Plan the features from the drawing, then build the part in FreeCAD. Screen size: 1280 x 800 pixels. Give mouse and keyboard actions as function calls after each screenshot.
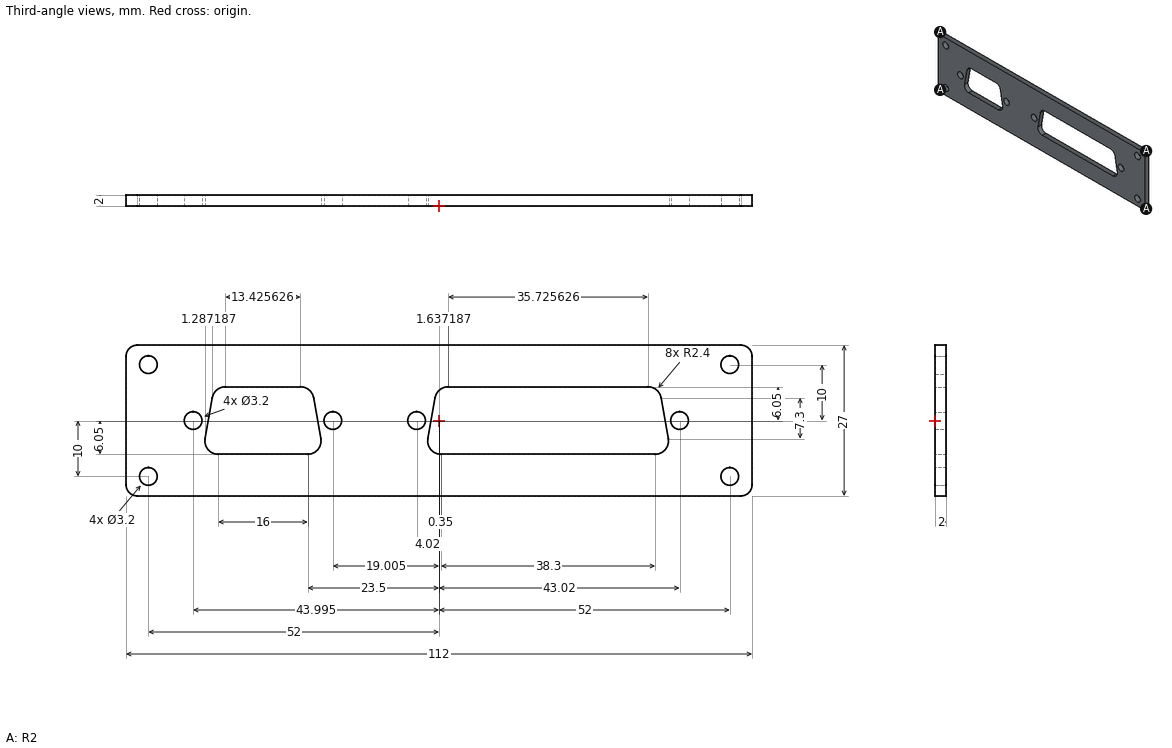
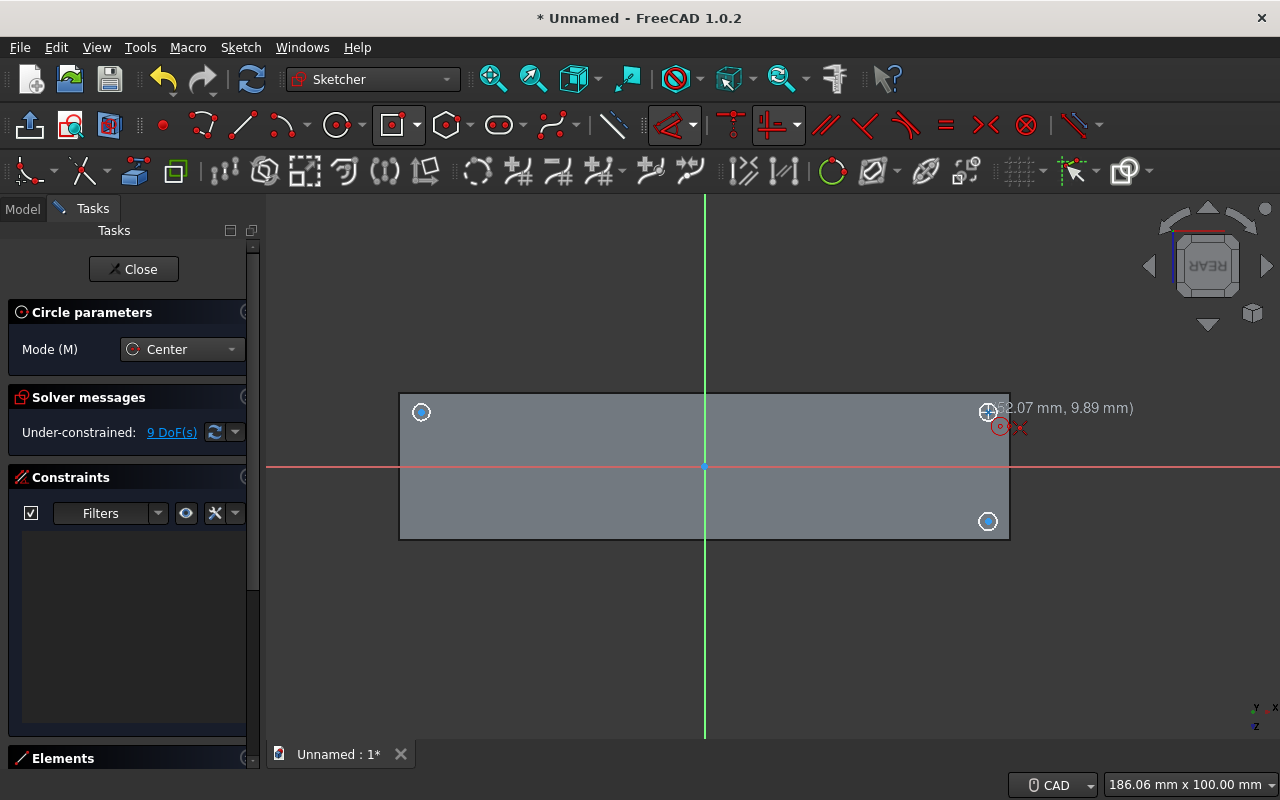
scroll(421, 521, up, 5)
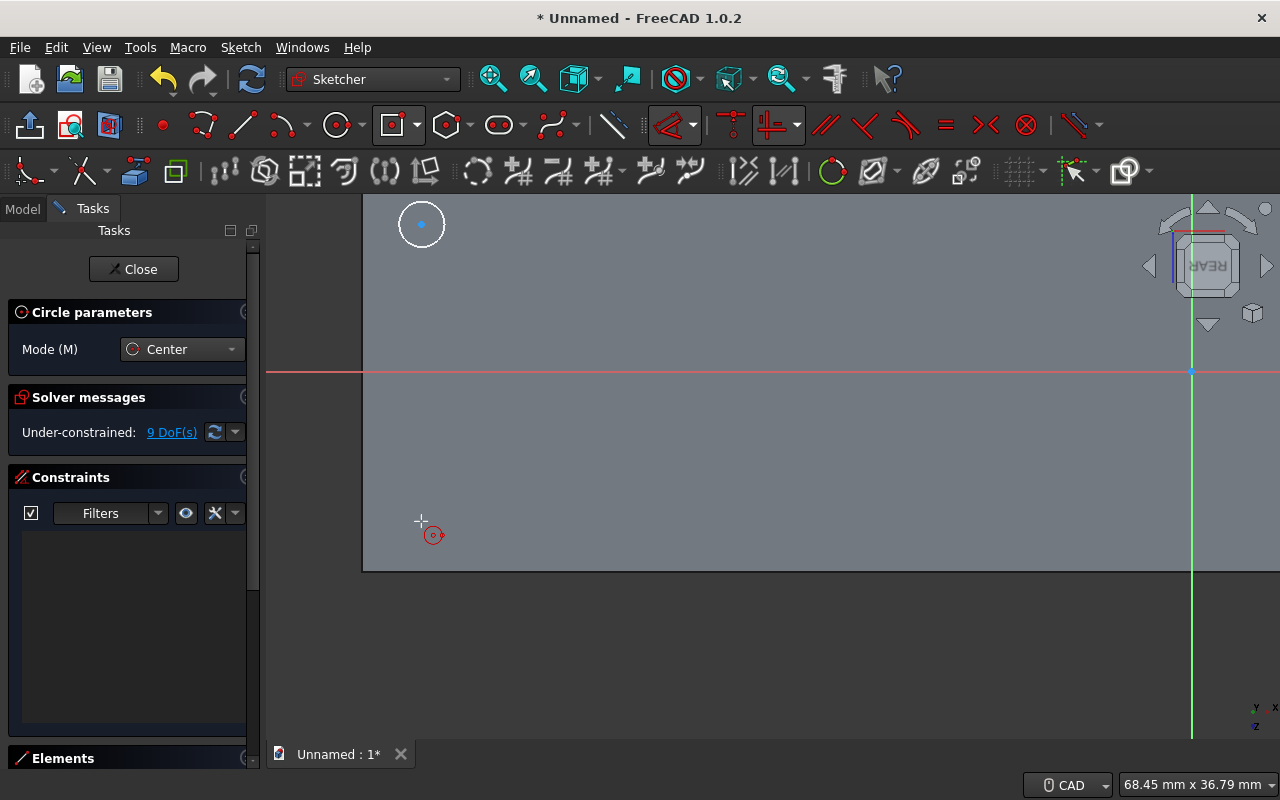
click(421, 520)
click(438, 503)
key(Escape)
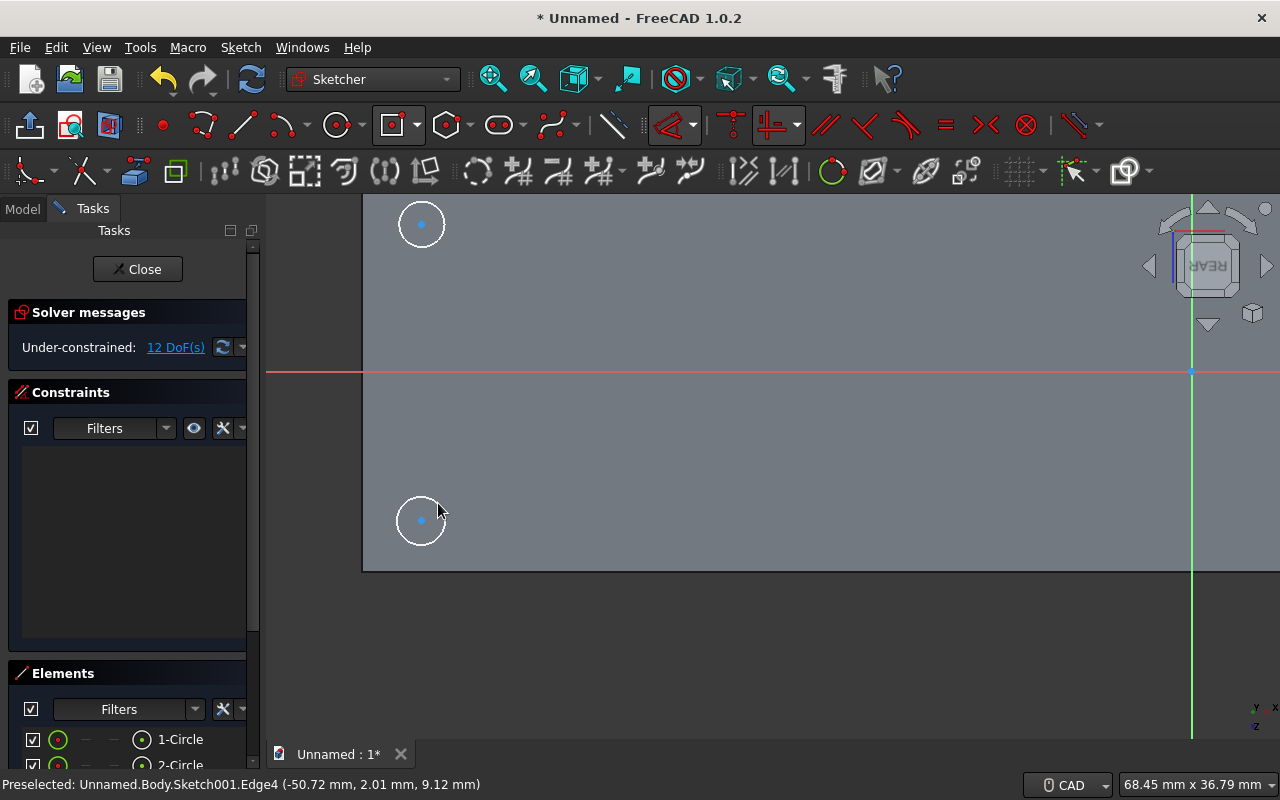
click(406, 240)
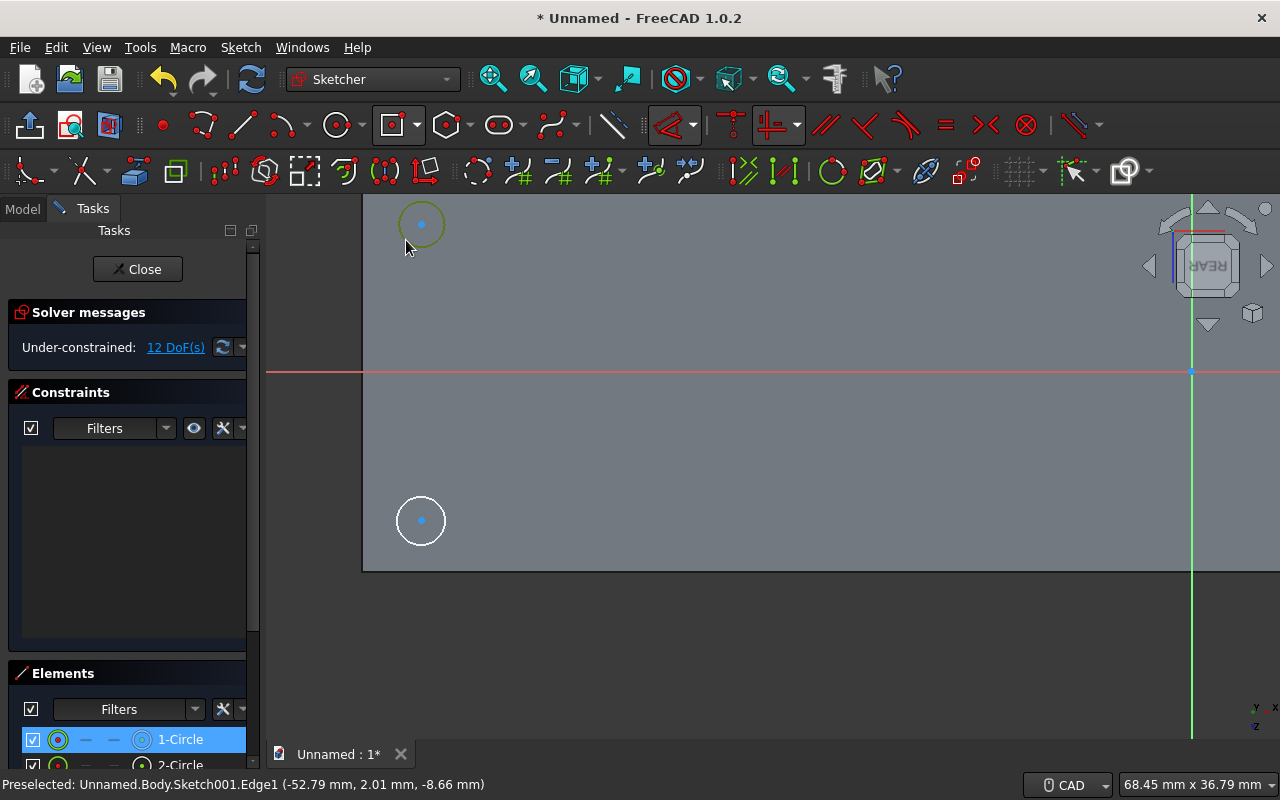
scroll(421, 522, down, 5)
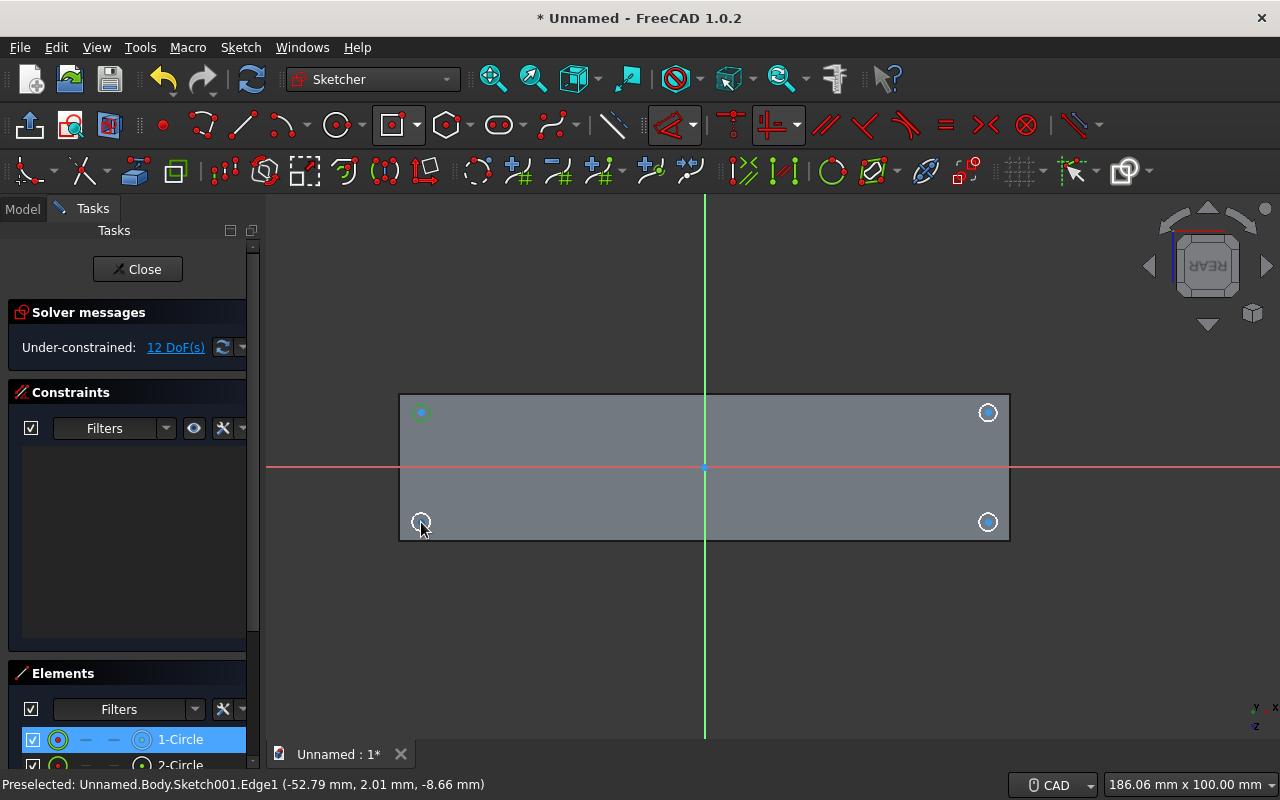
scroll(994, 407, up, 3)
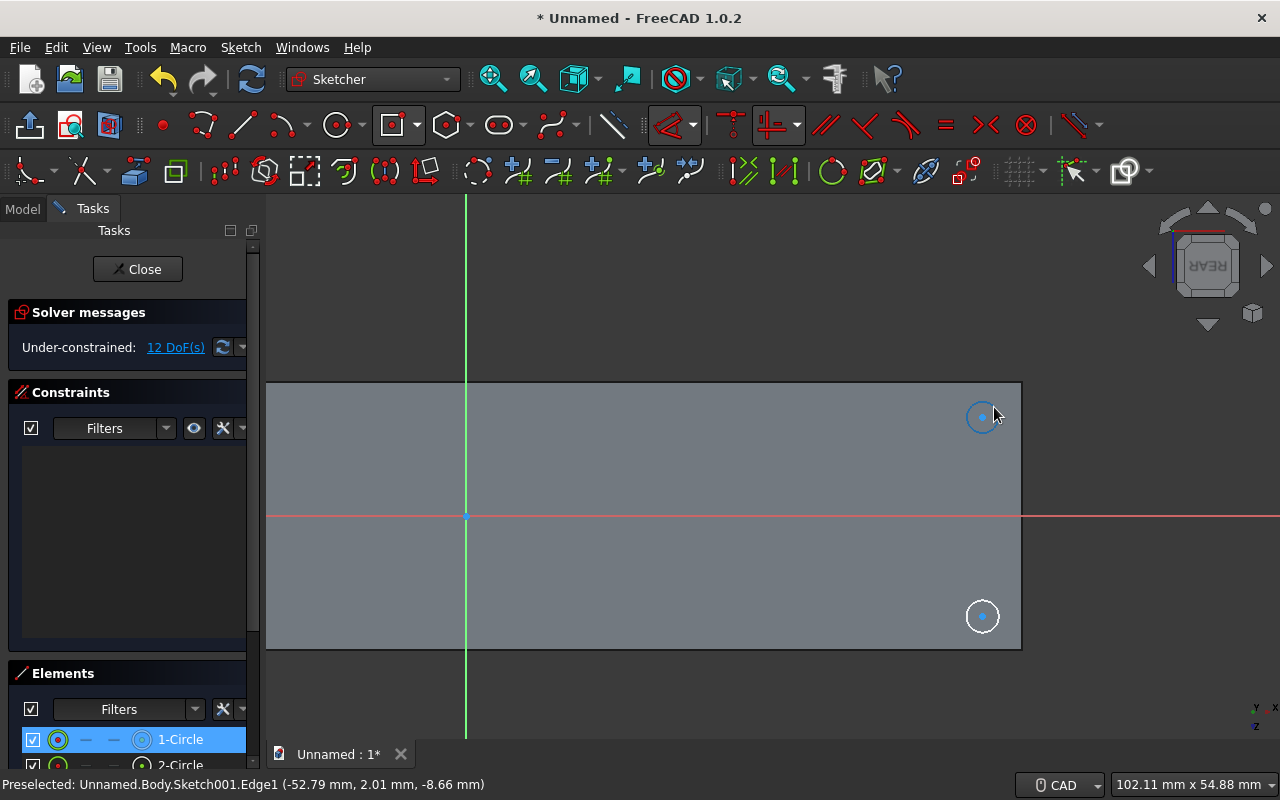
click(994, 406)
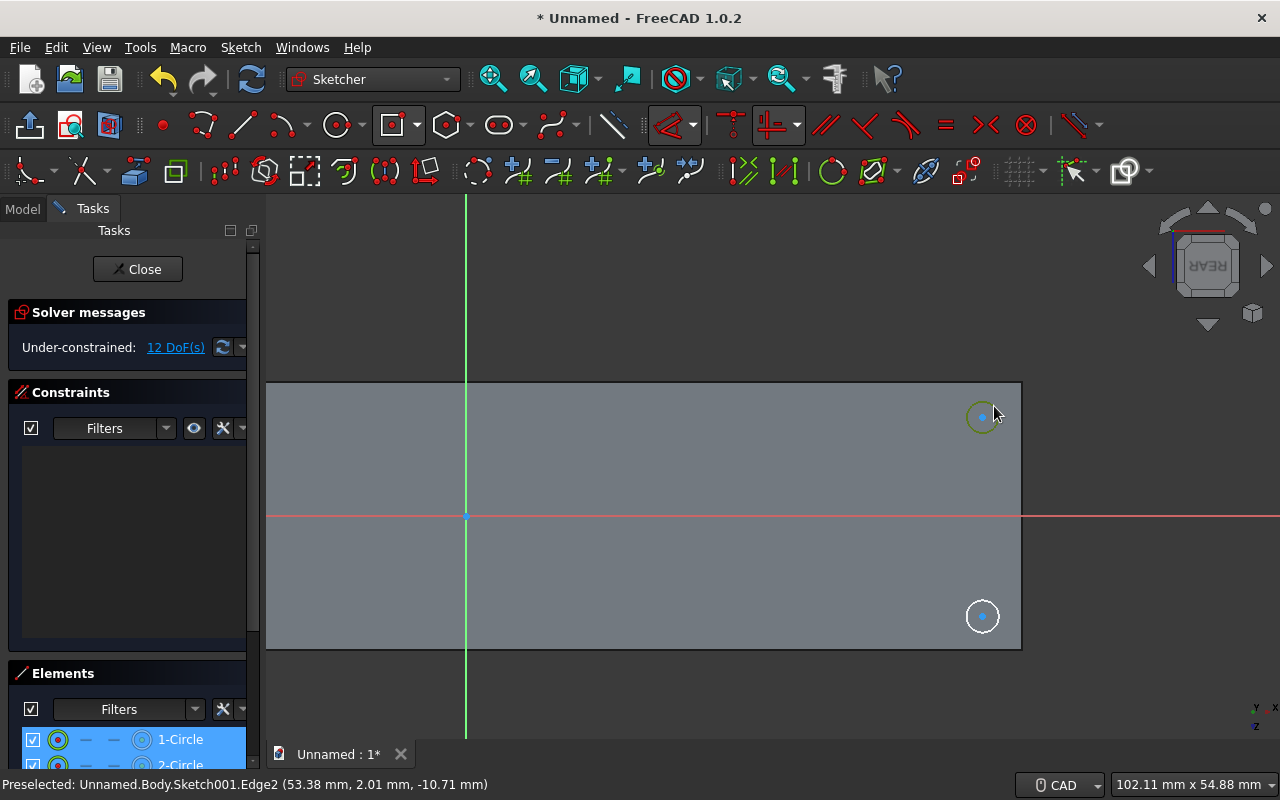
click(994, 605)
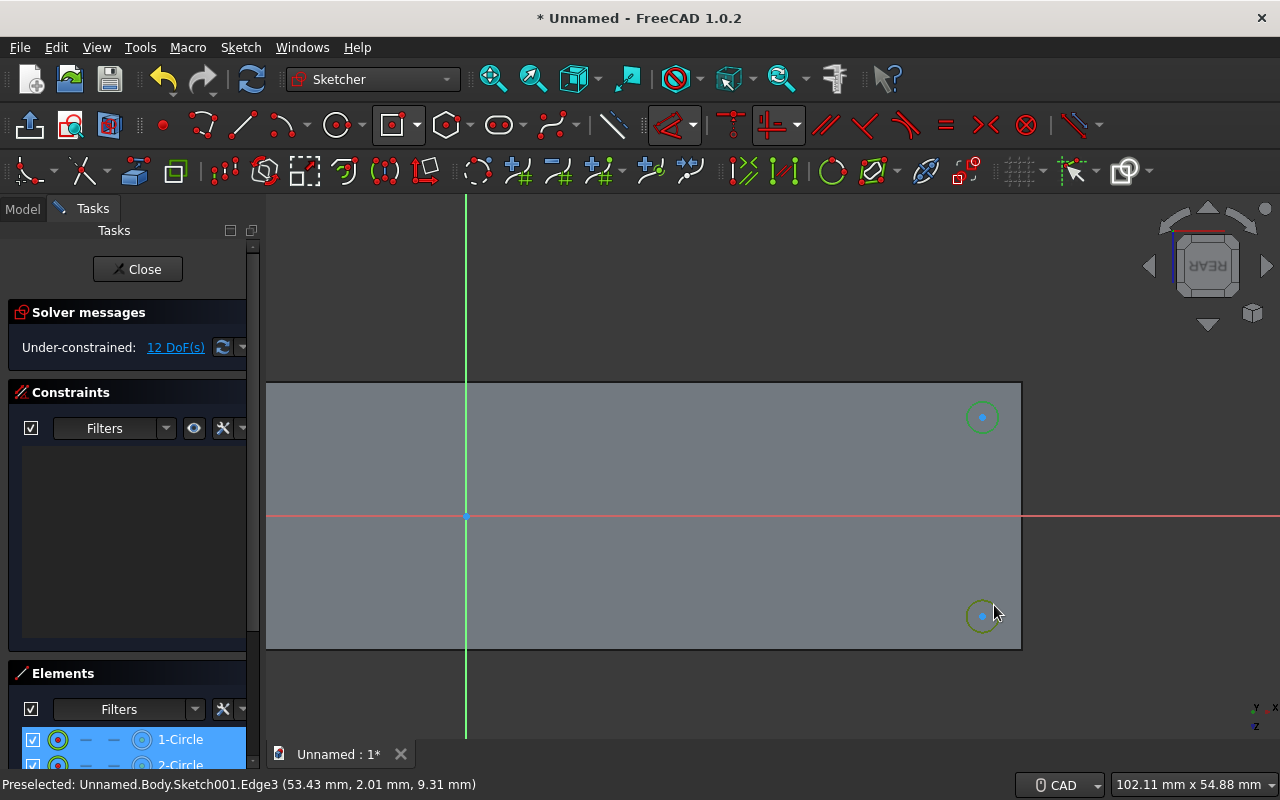
scroll(994, 406, down, 3)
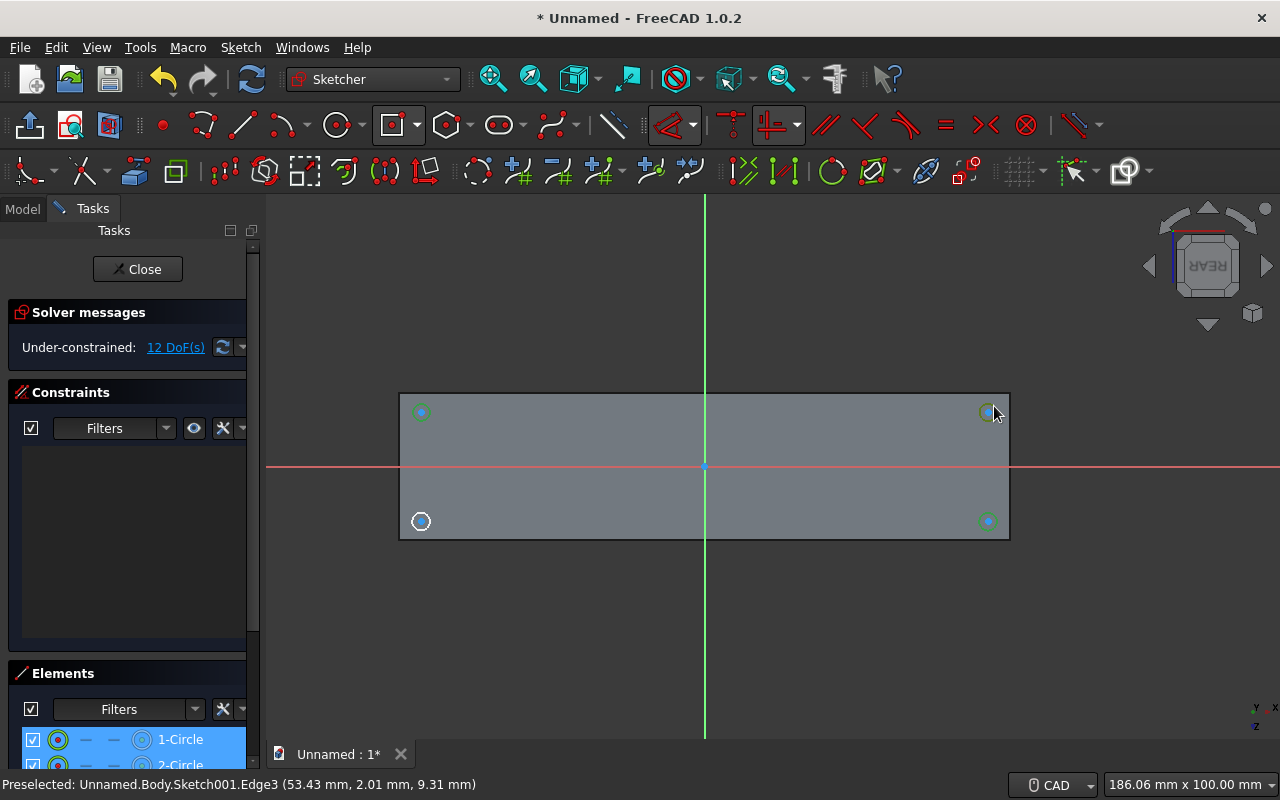
scroll(427, 515, up, 3)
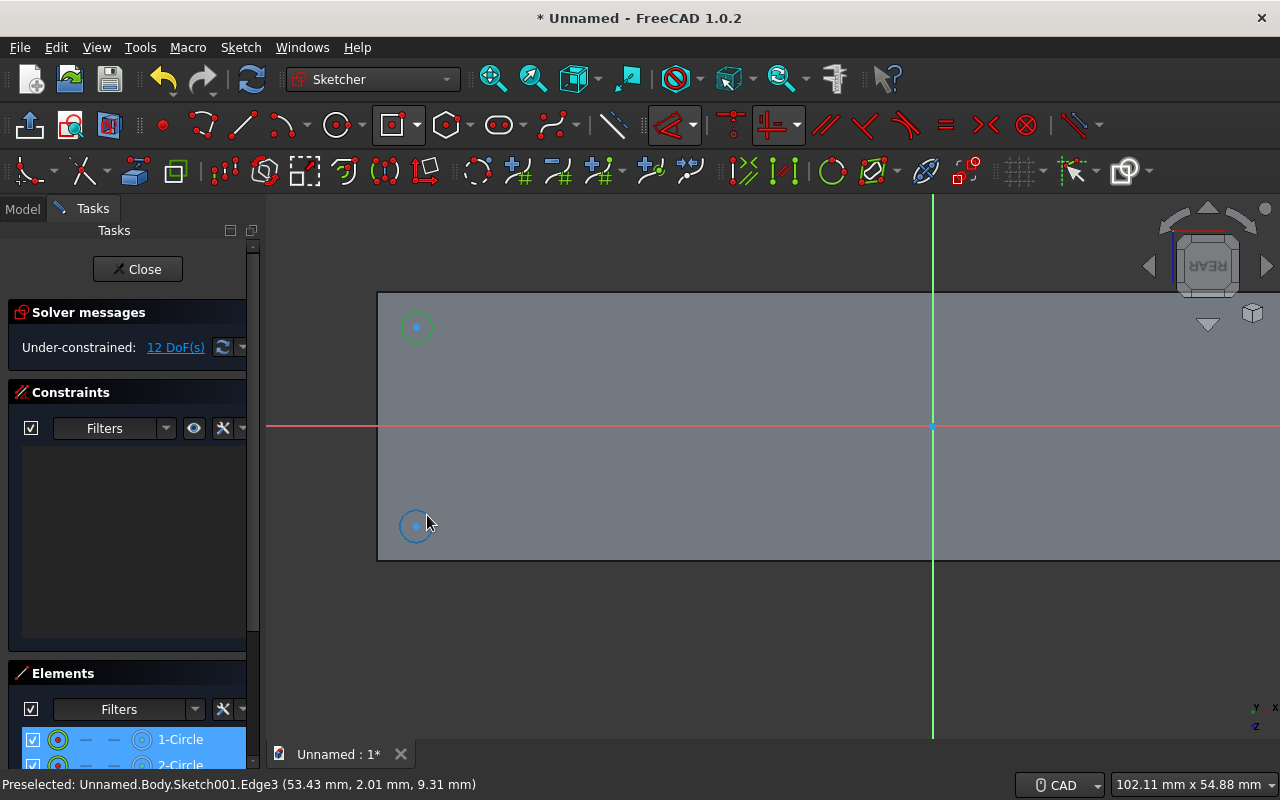
click(427, 515)